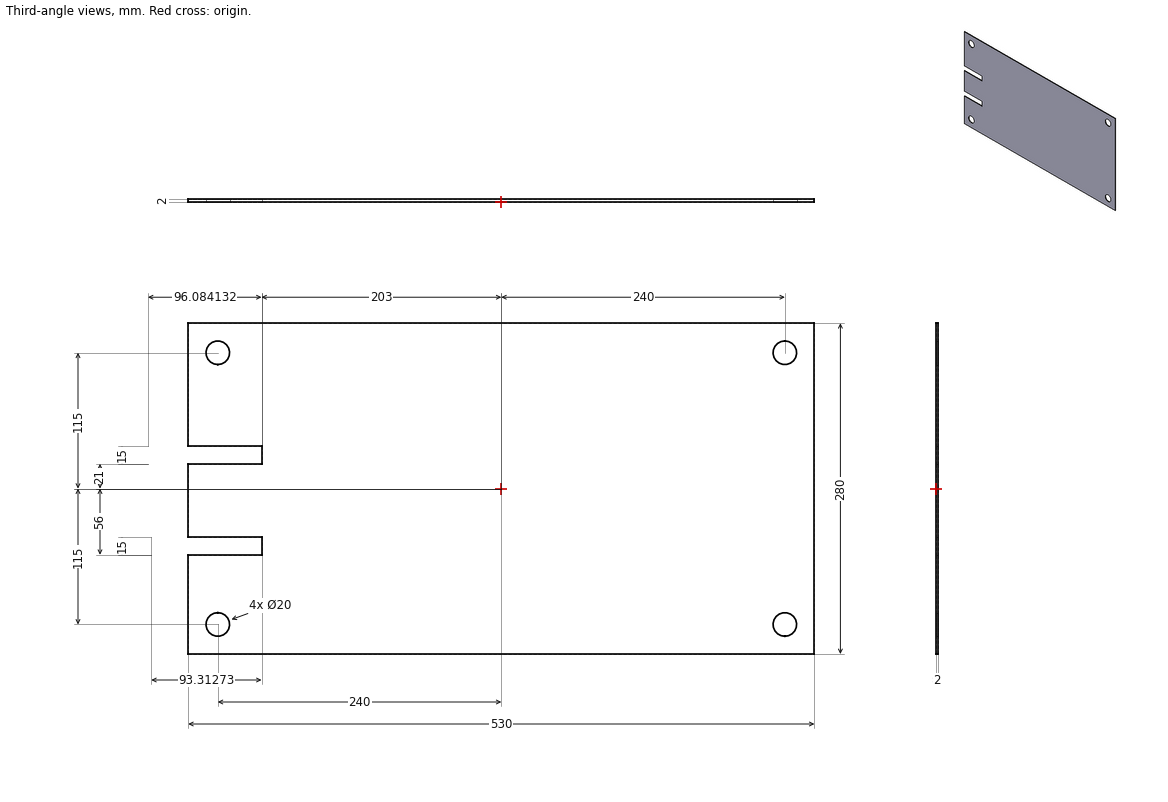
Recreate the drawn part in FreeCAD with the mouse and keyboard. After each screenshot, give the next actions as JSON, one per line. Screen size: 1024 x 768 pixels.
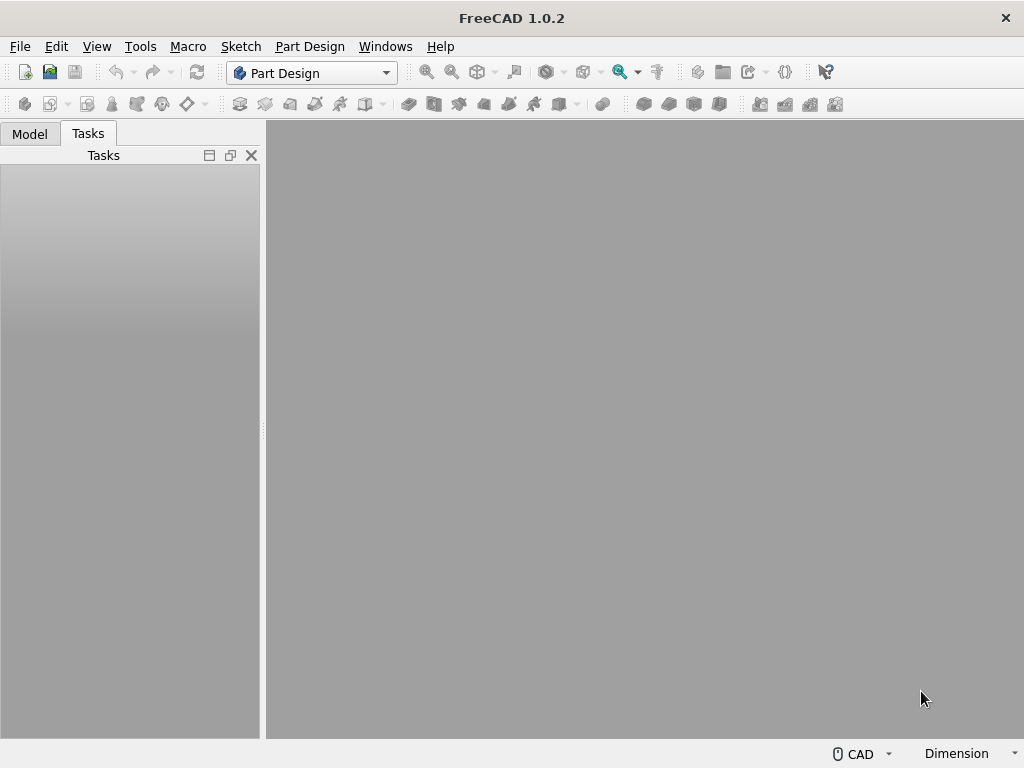
{"action": "left_click", "coordinate": [25, 72]}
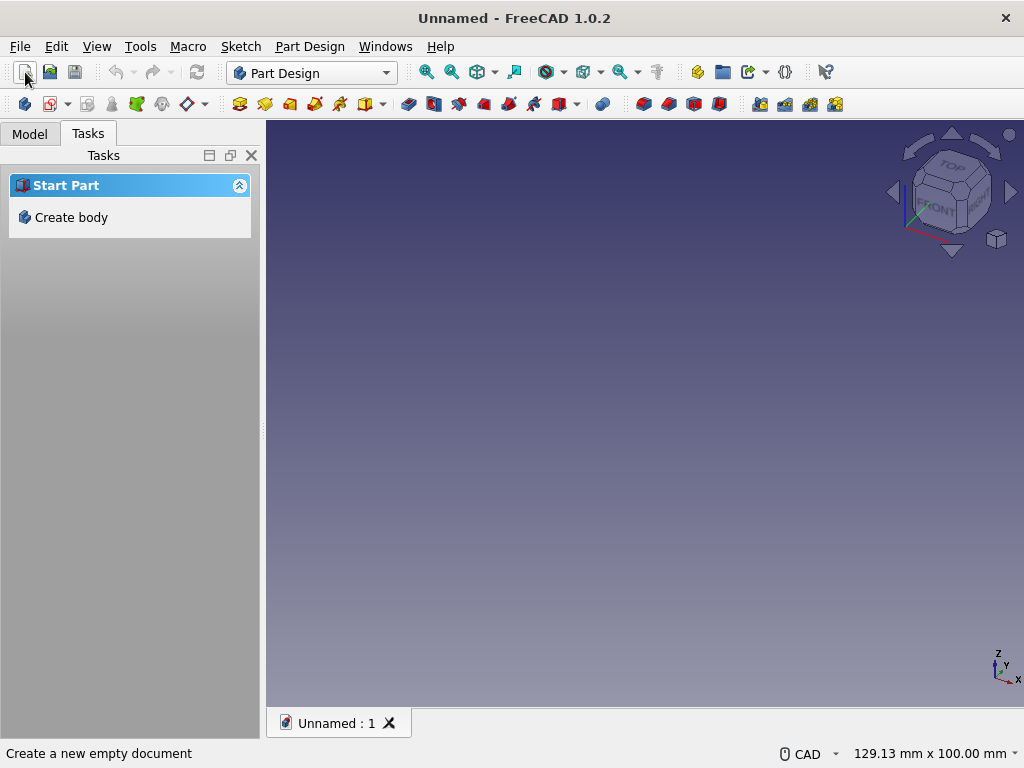
{"action": "left_click", "coordinate": [50, 104]}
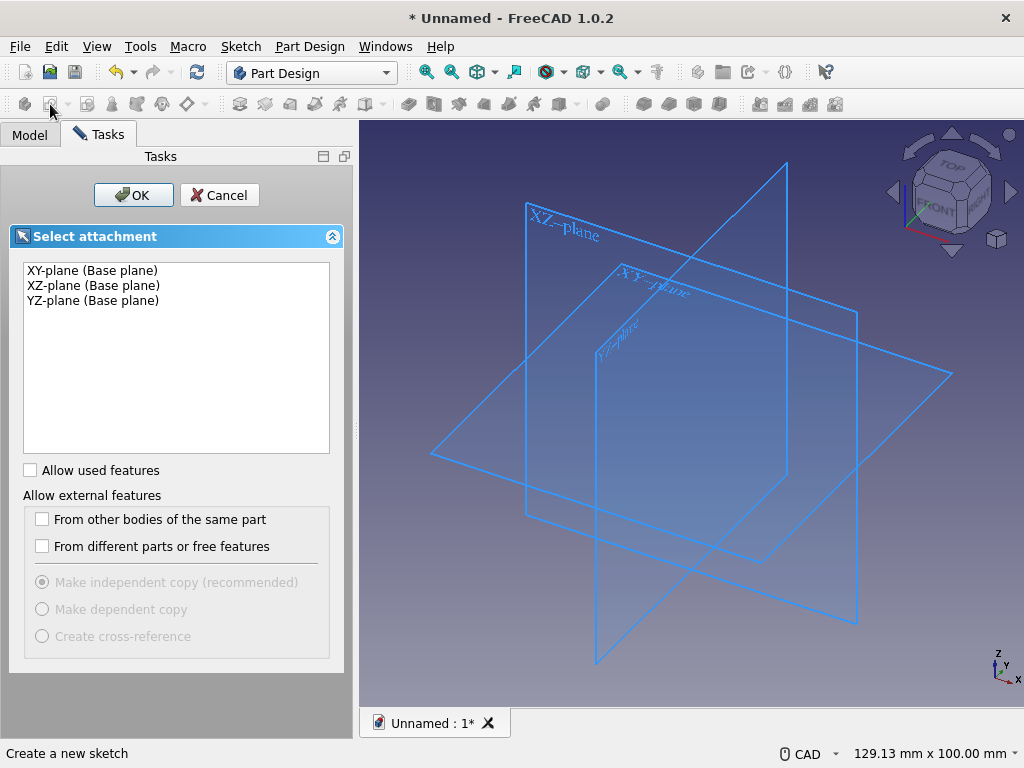
{"action": "left_click", "coordinate": [84, 286]}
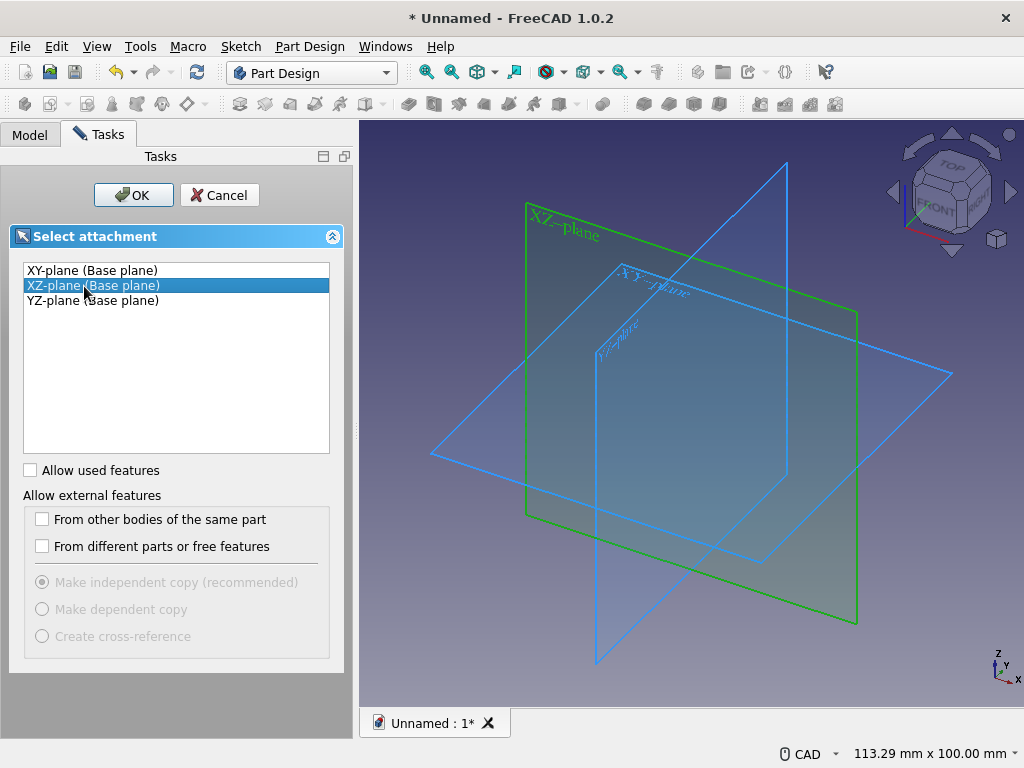
{"action": "left_click", "coordinate": [134, 195]}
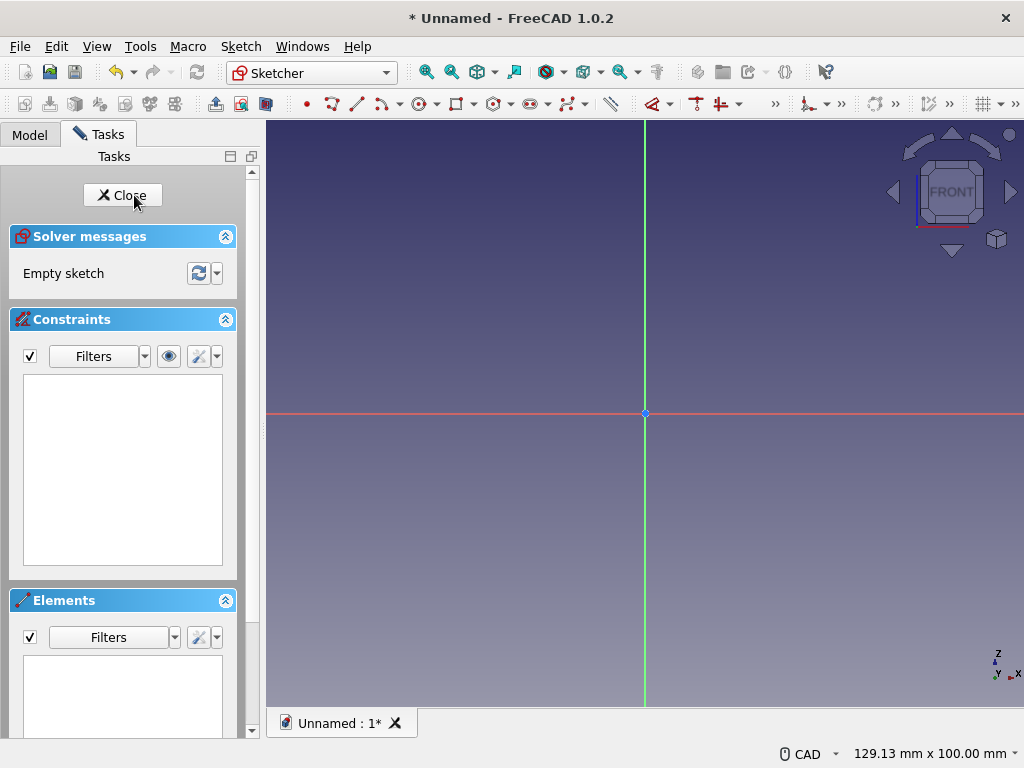
{"action": "scroll", "coordinate": [566, 414], "scroll_direction": "down", "scroll_amount": 10}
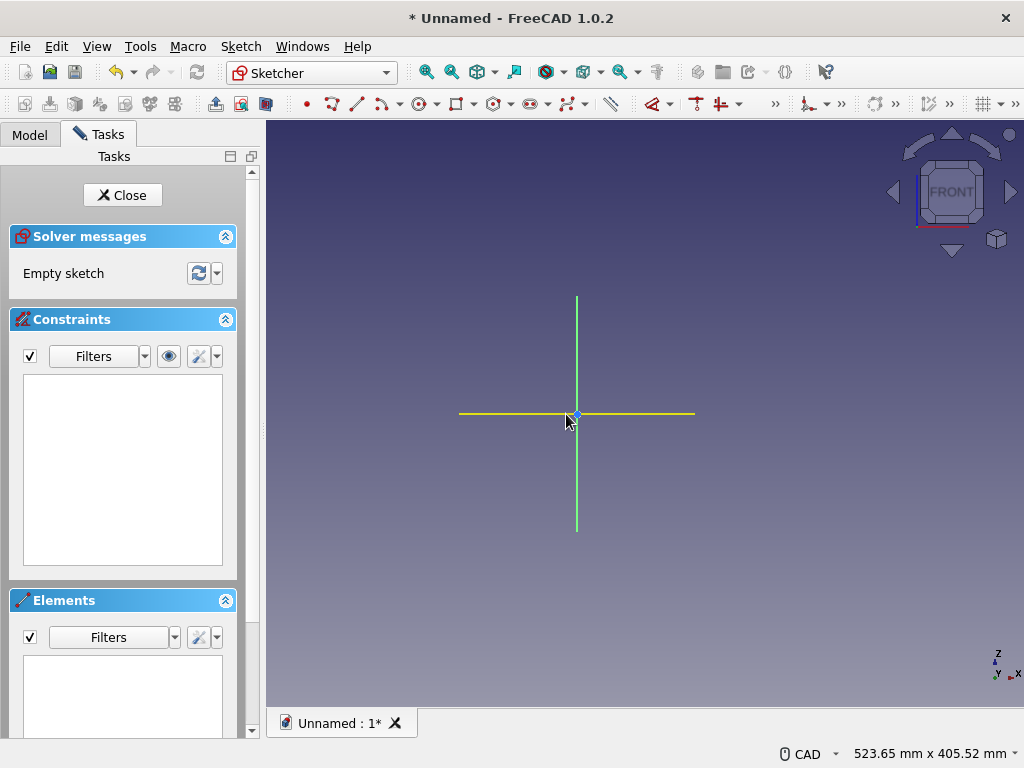
{"action": "left_click", "coordinate": [474, 104]}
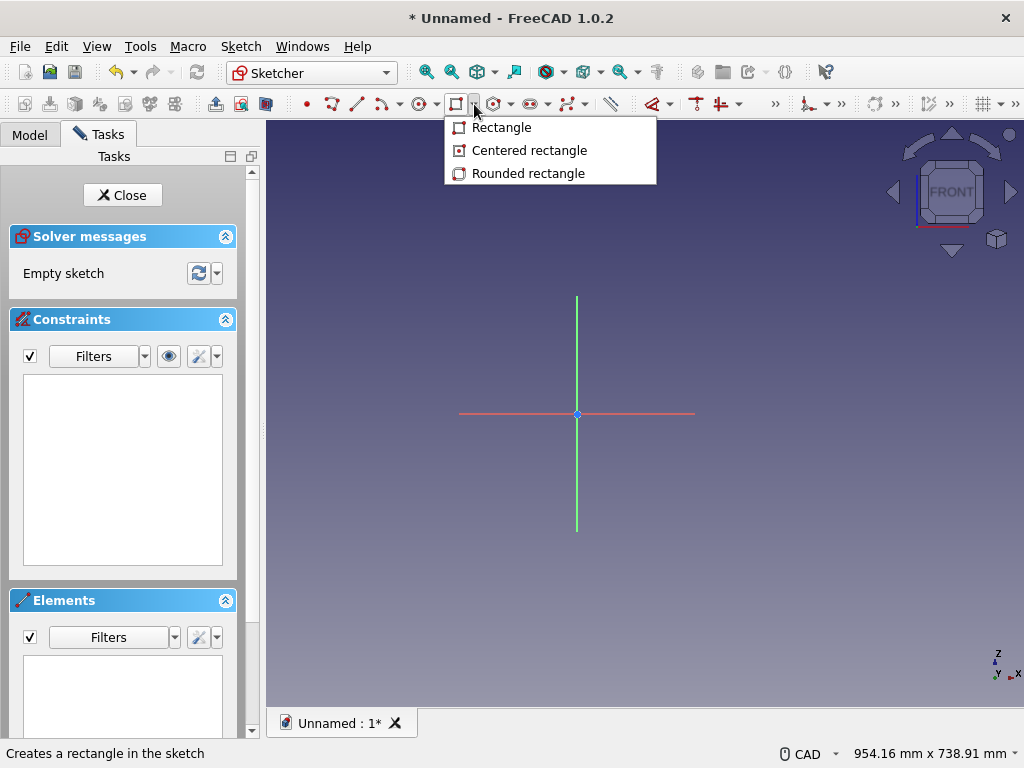
{"action": "left_click", "coordinate": [550, 150]}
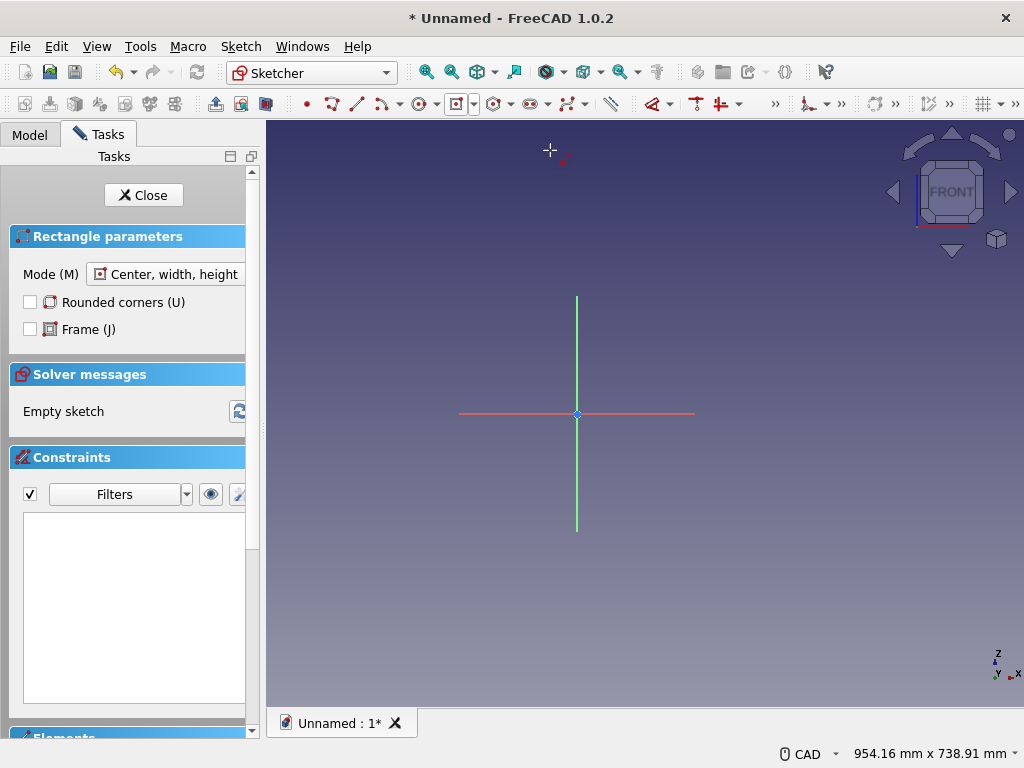
{"action": "left_click", "coordinate": [577, 414]}
{"action": "left_click", "coordinate": [788, 303]}
{"action": "key", "text": "Escape"}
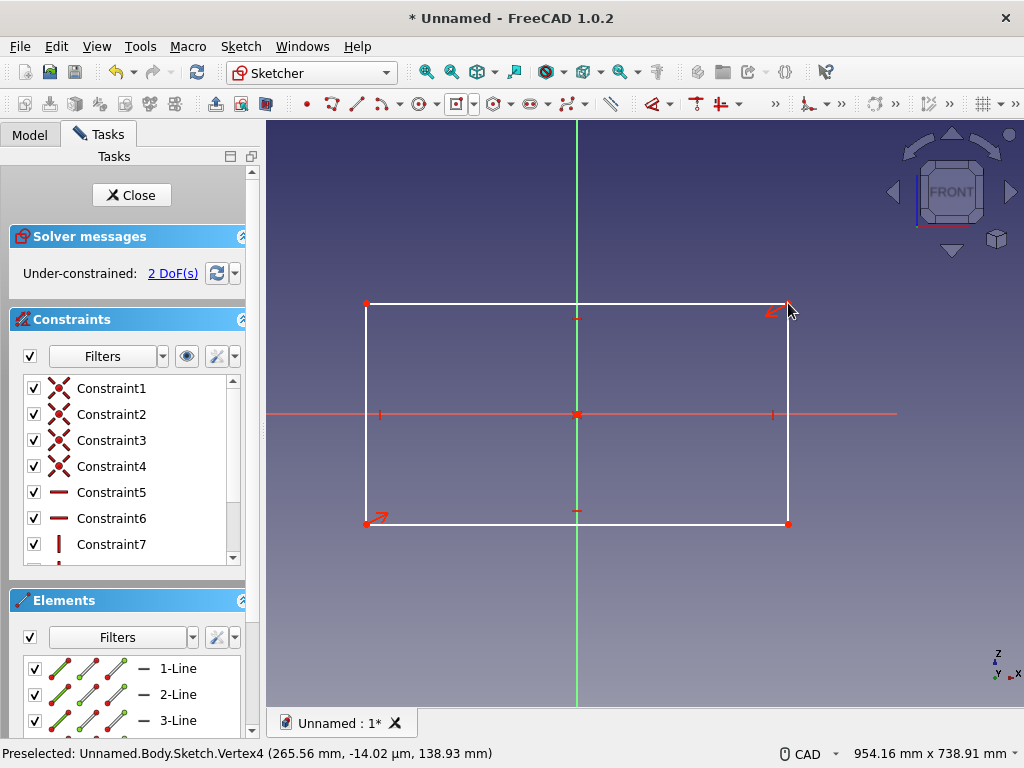
{"action": "left_click", "coordinate": [652, 104]}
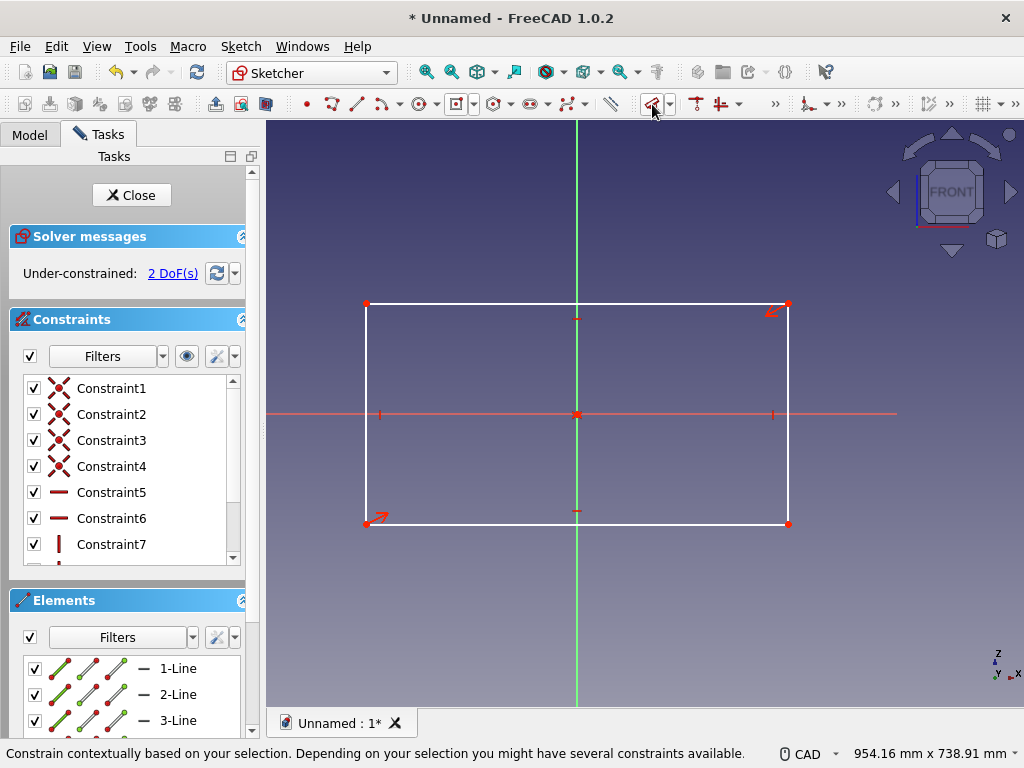
{"action": "left_click", "coordinate": [493, 525]}
{"action": "left_click", "coordinate": [480, 559]}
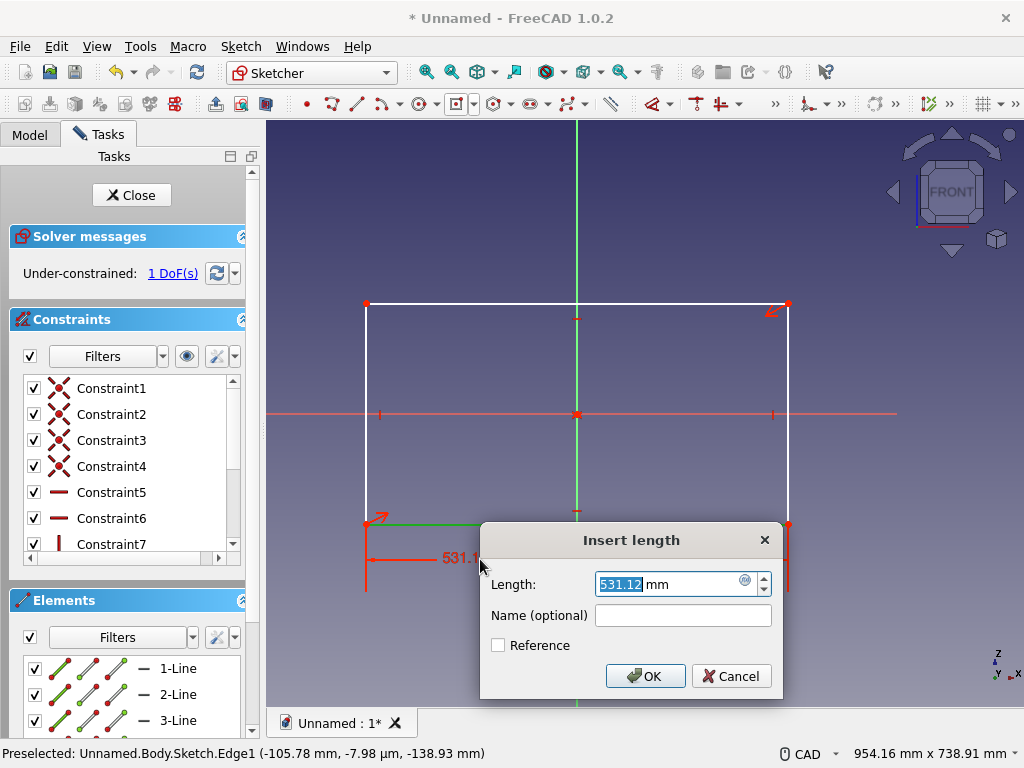
{"action": "type", "text": "530"}
{"action": "key", "text": "Return"}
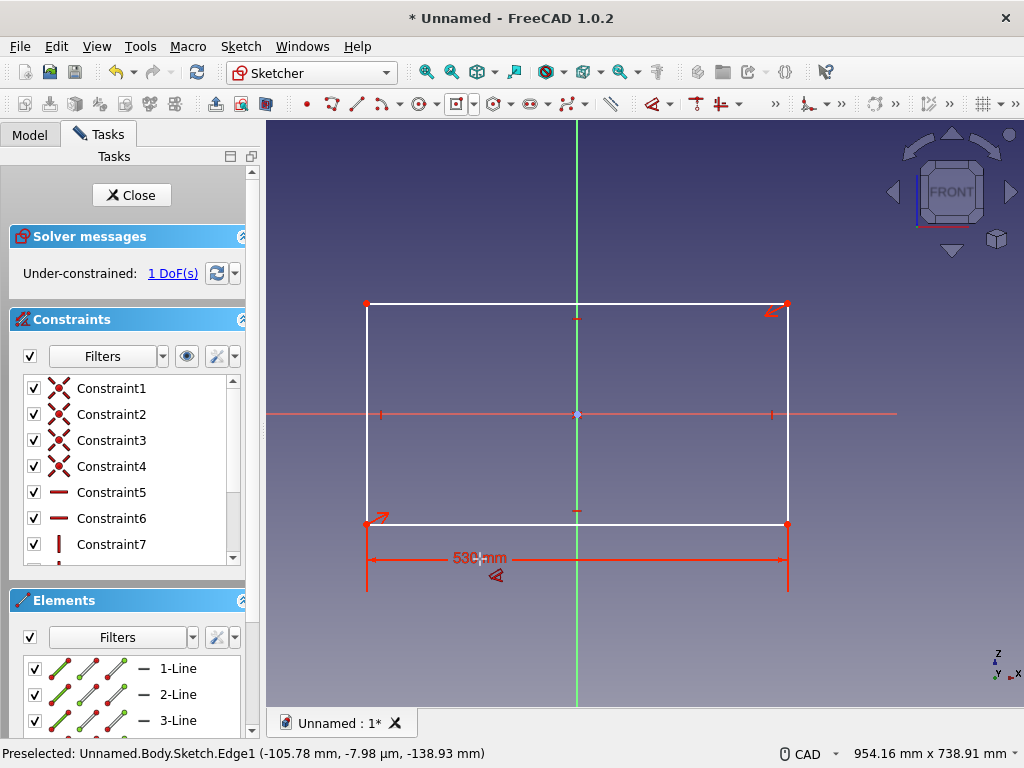
{"action": "left_click", "coordinate": [788, 459]}
{"action": "left_click", "coordinate": [822, 364]}